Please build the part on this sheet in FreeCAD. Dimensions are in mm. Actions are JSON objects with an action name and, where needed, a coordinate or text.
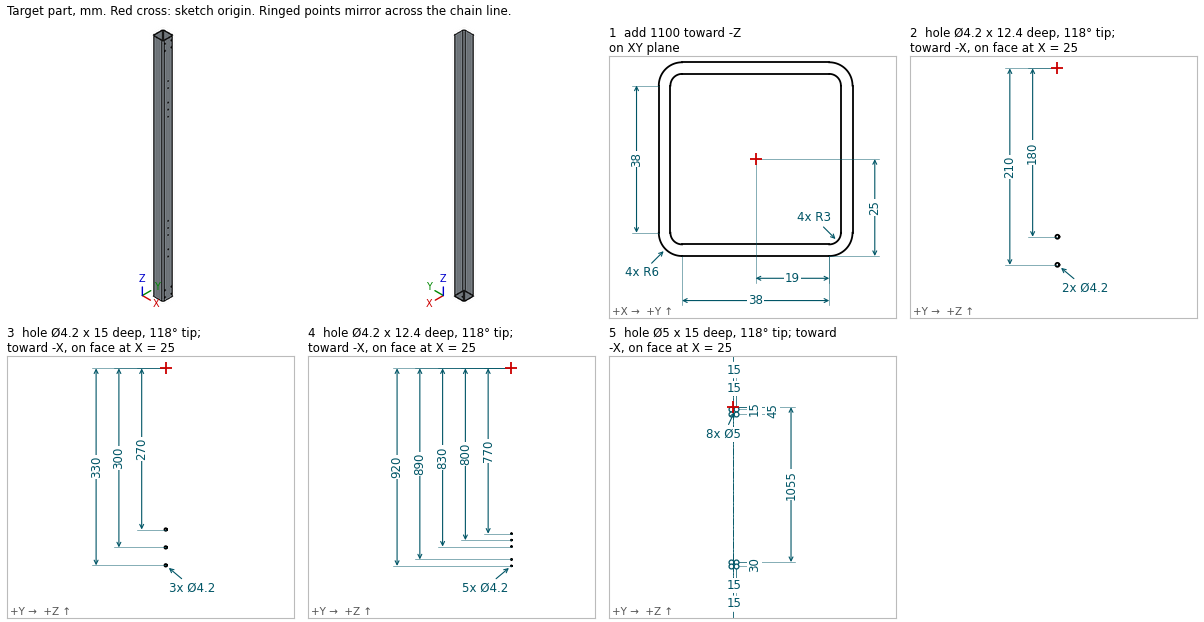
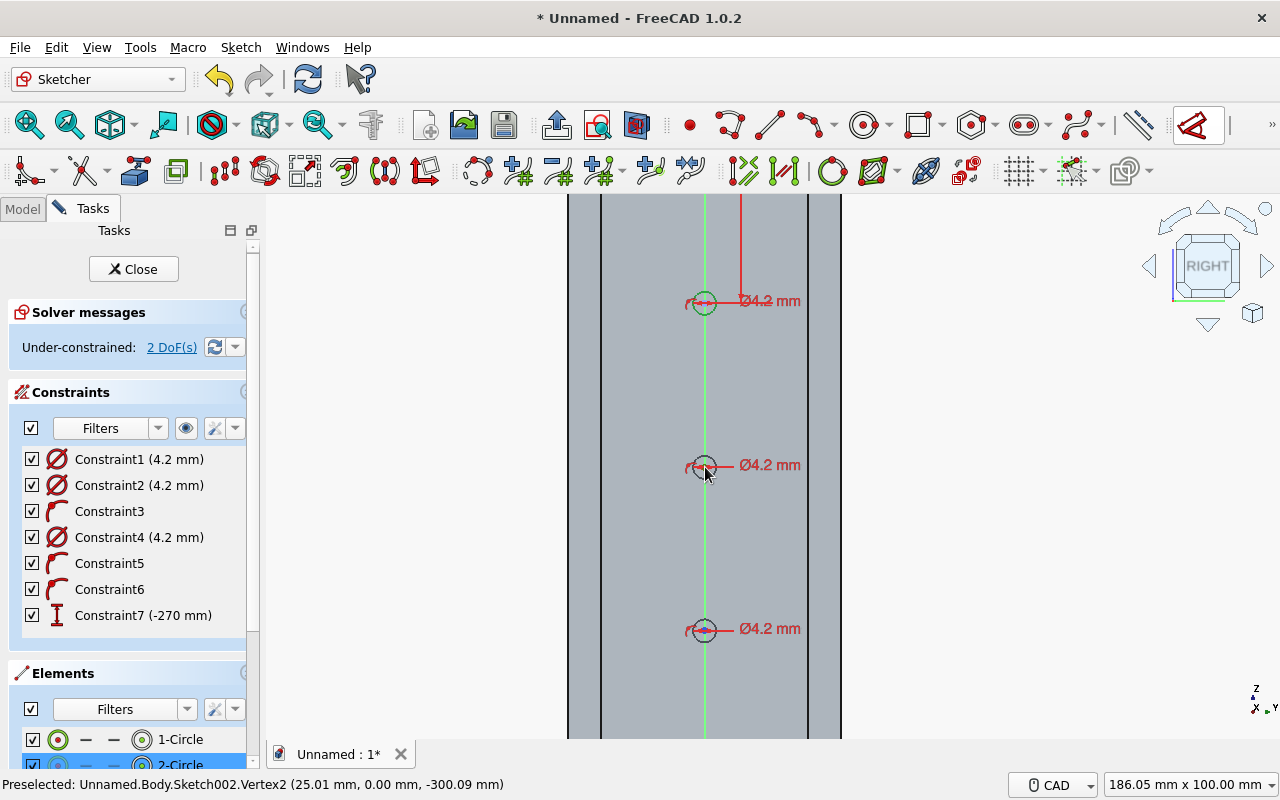
{"action": "key", "text": "i"}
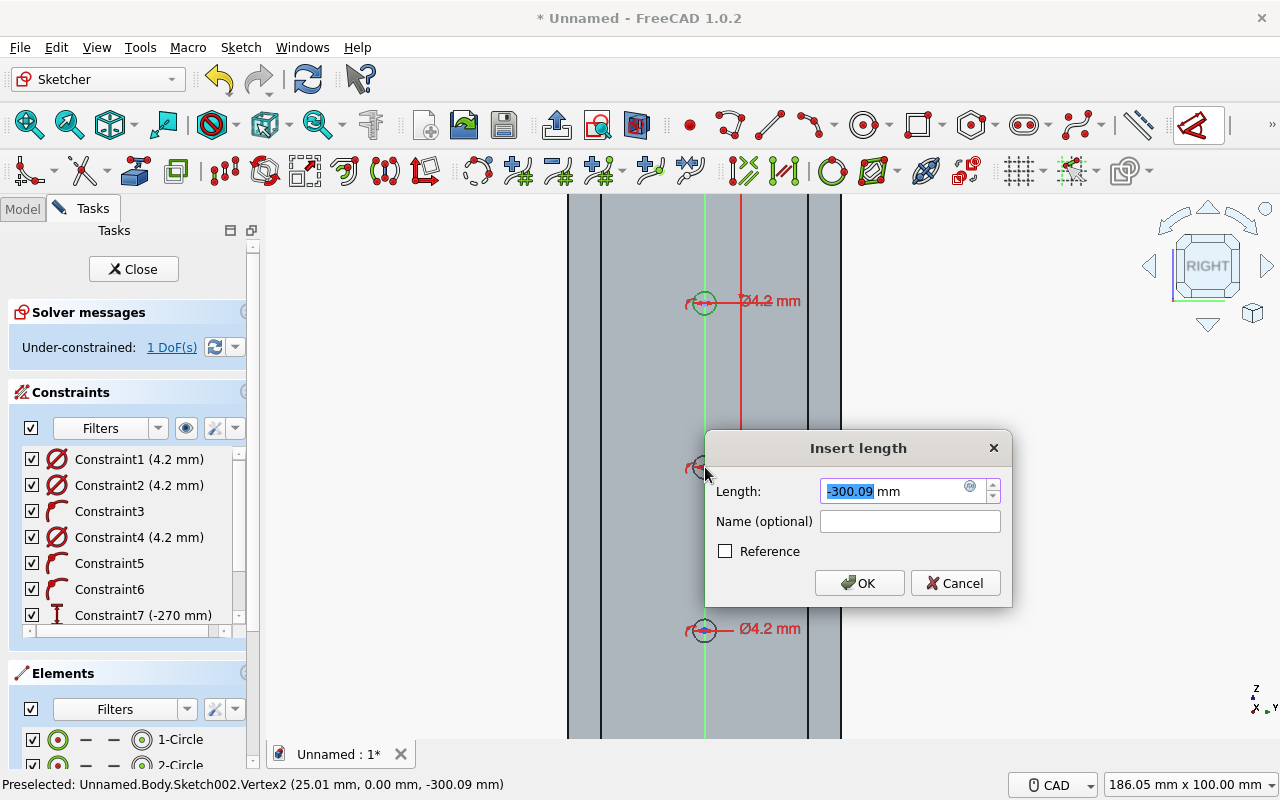
{"action": "type", "text": "-300"}
{"action": "key", "text": "Return"}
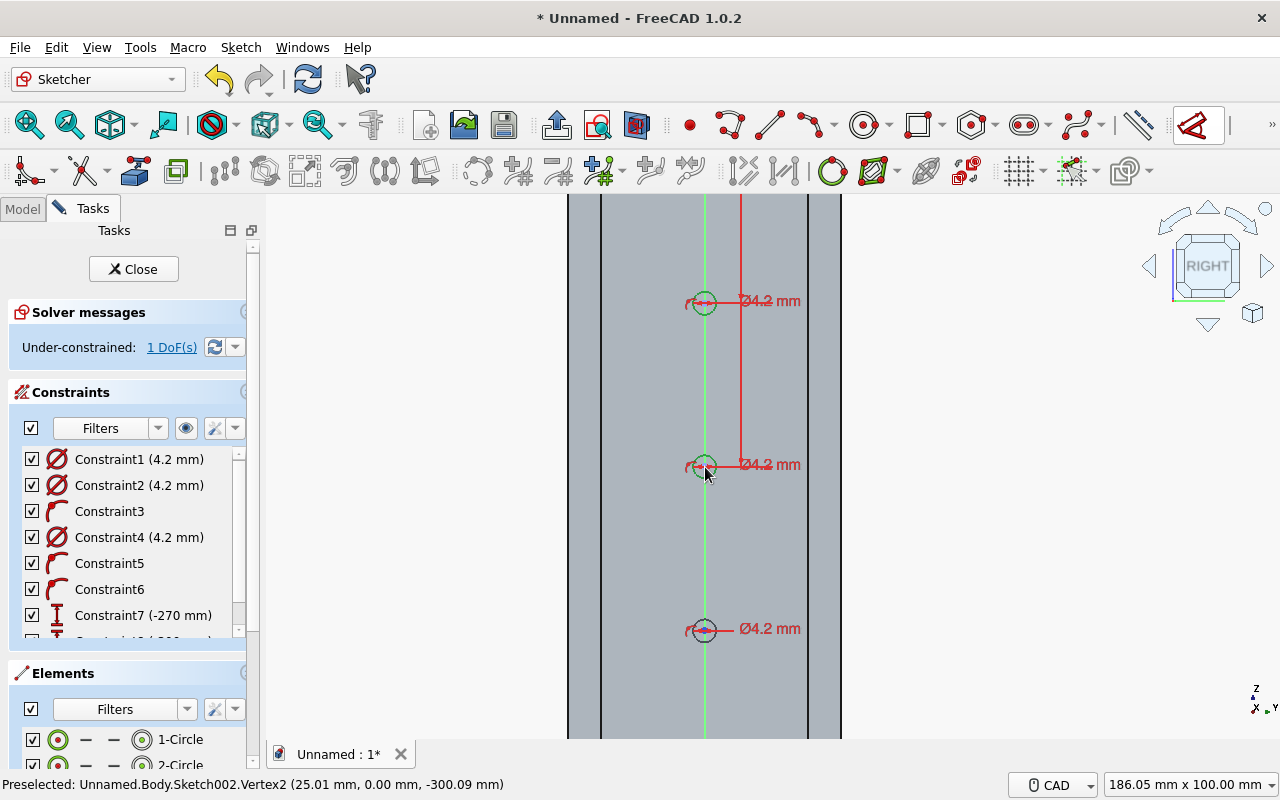
{"action": "left_click", "coordinate": [705, 631]}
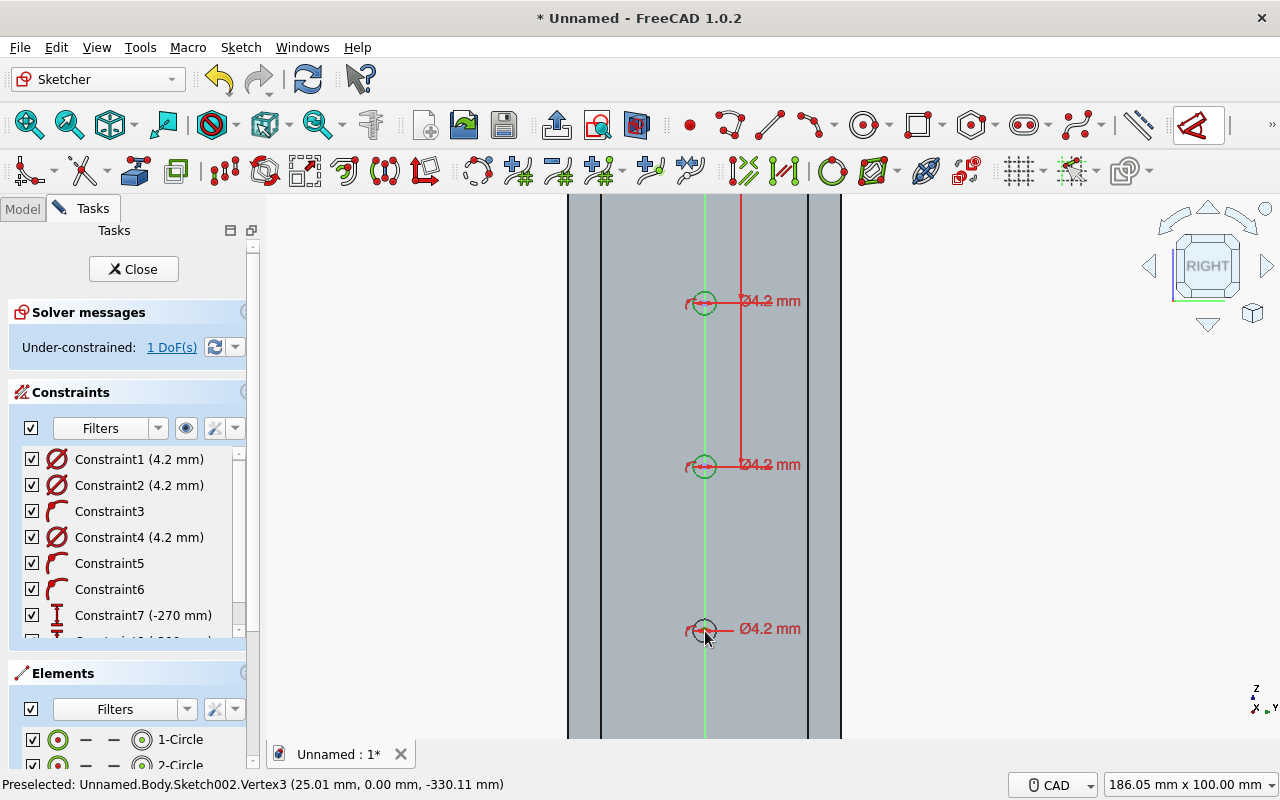
{"action": "left_click", "coordinate": [1218, 126]}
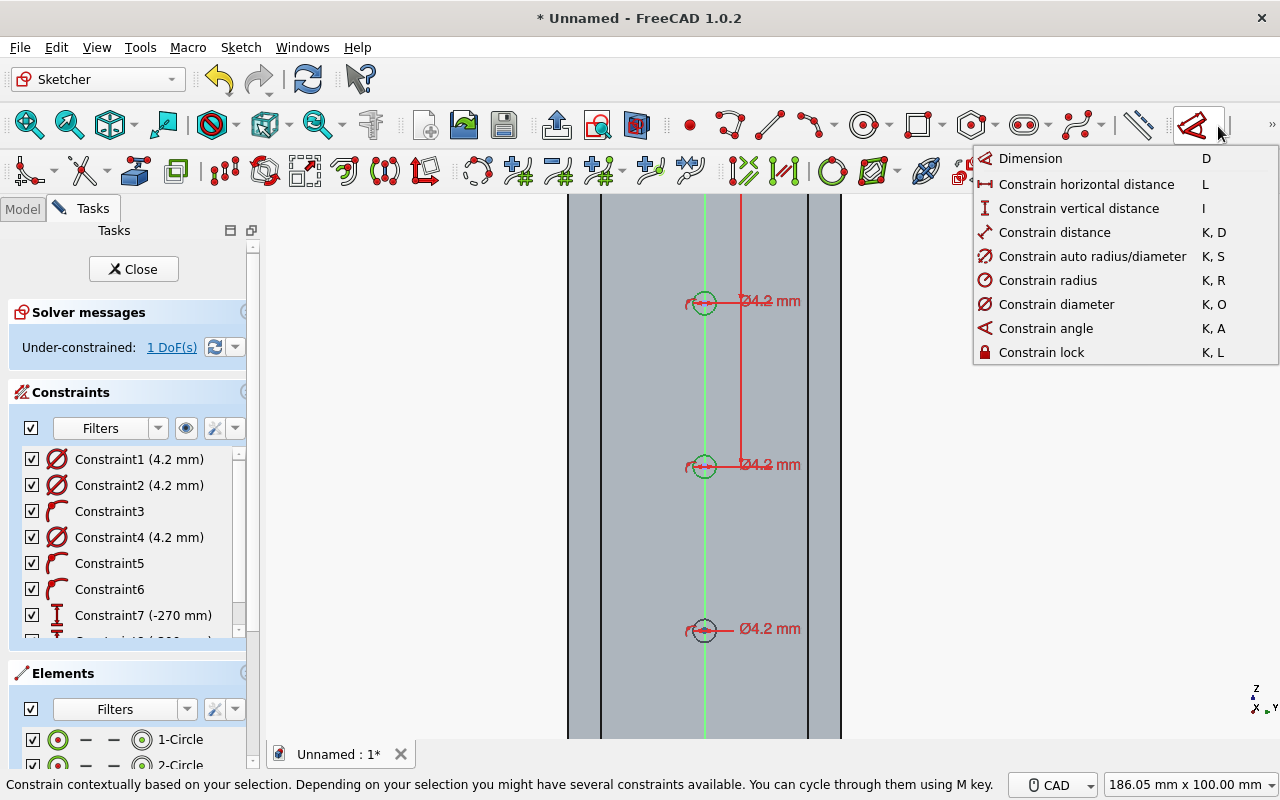
{"action": "left_click", "coordinate": [1126, 208]}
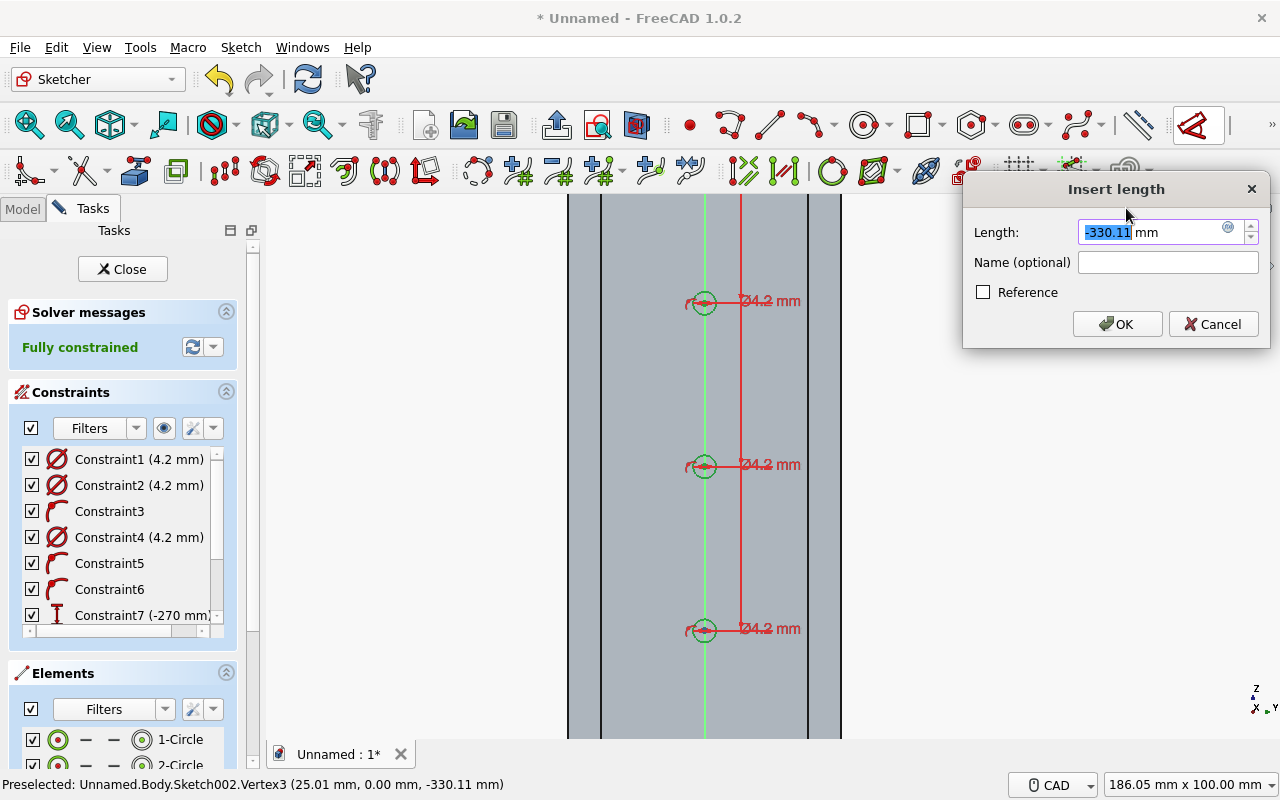
{"action": "type", "text": "-330"}
{"action": "key", "text": "Return"}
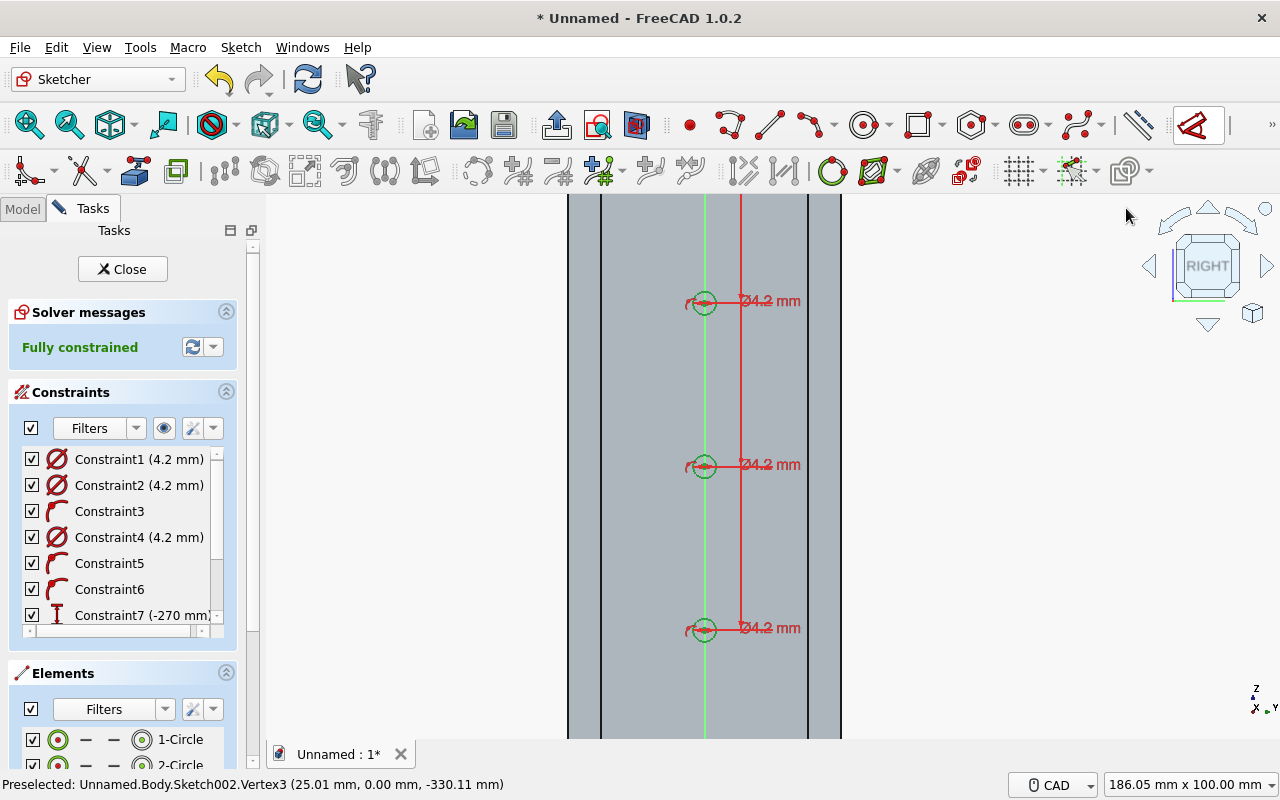
{"action": "left_click", "coordinate": [123, 269]}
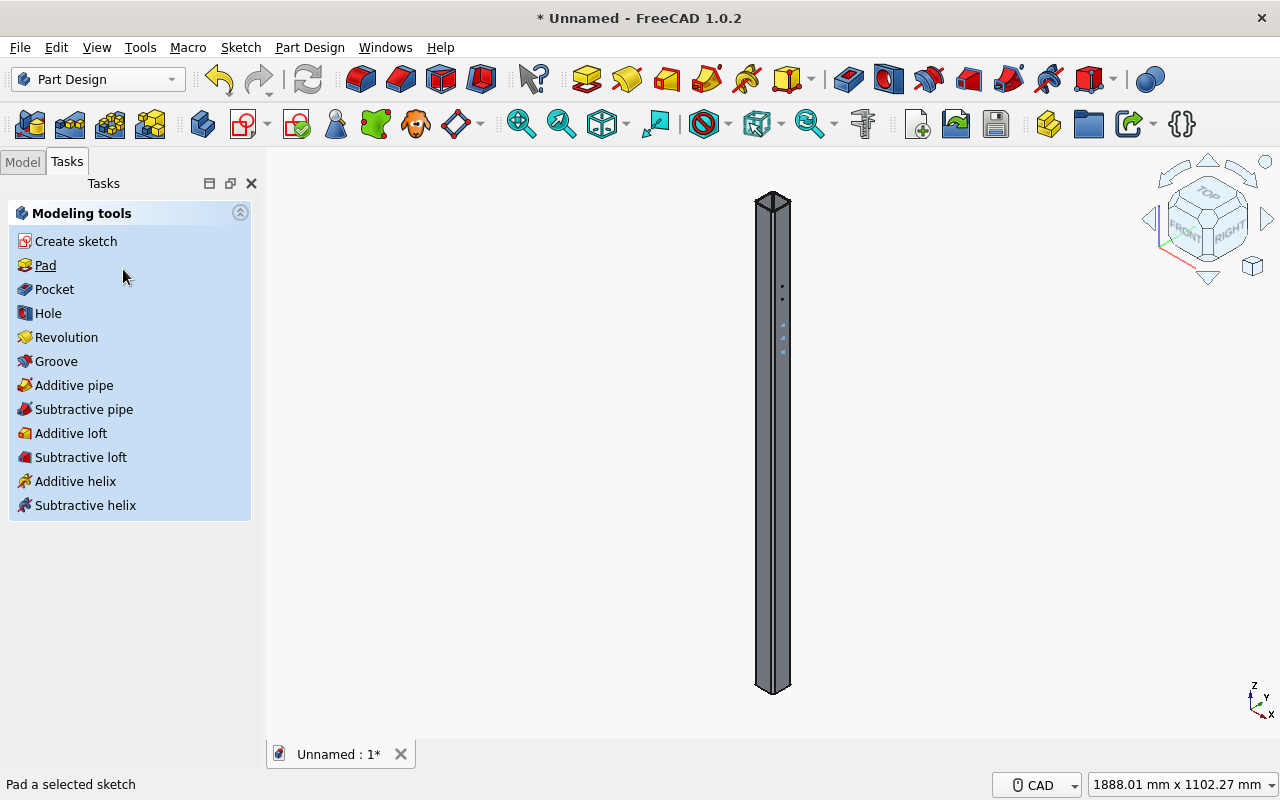
{"action": "left_click", "coordinate": [890, 80]}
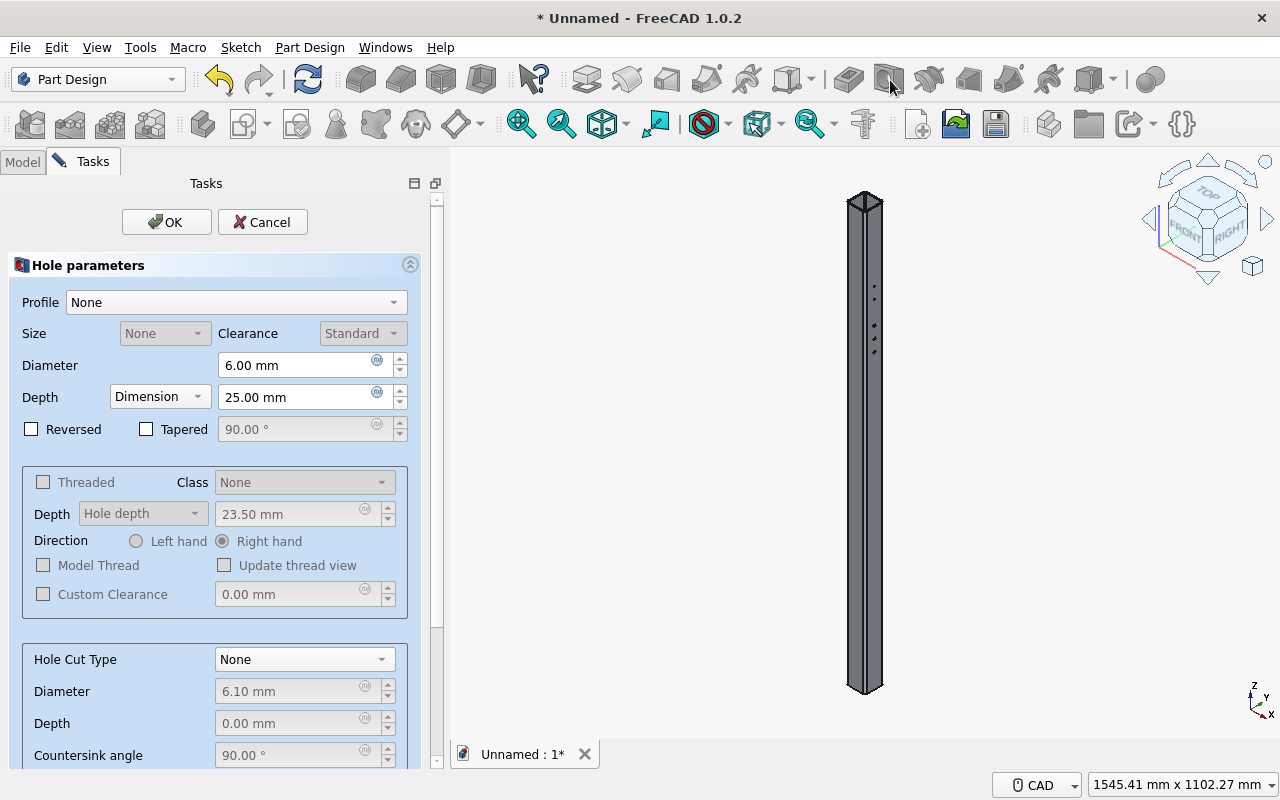
{"action": "triple_click", "coordinate": [305, 365]}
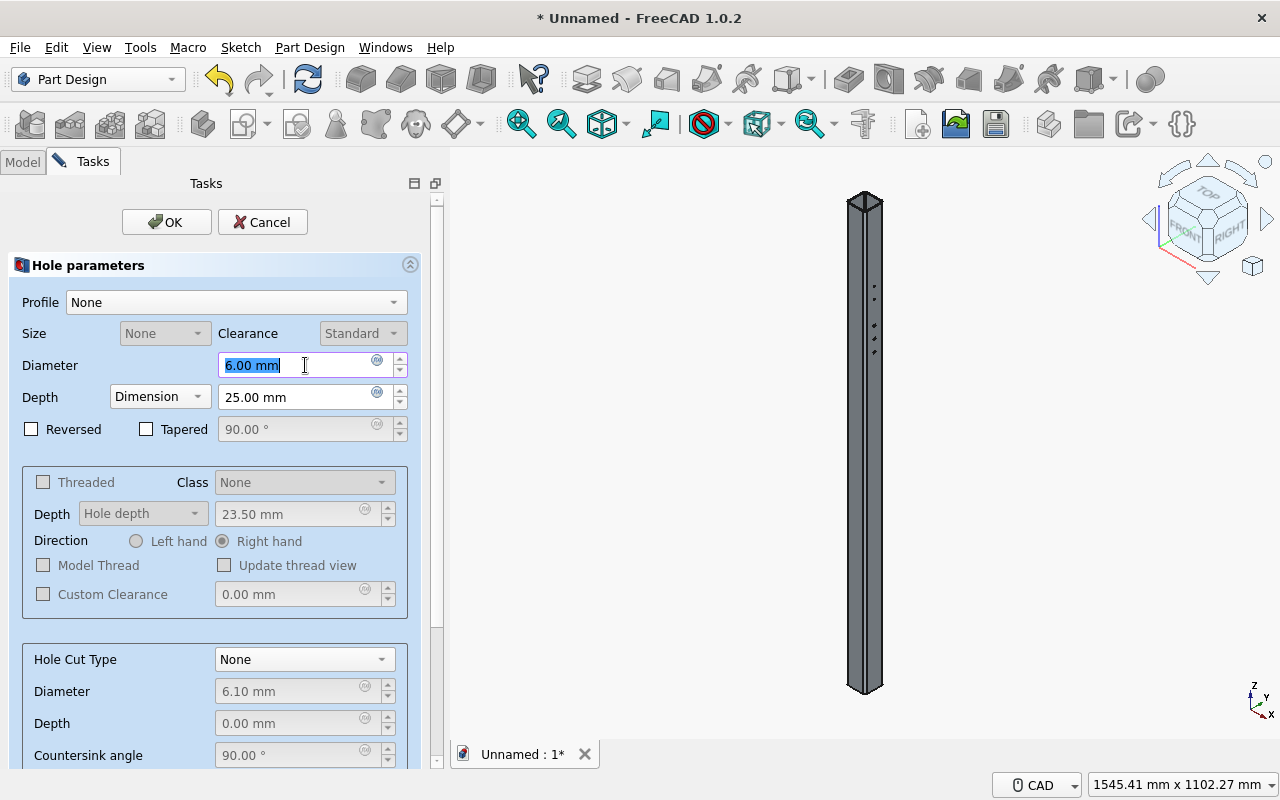
{"action": "type", "text": "4.2"}
{"action": "key", "text": "Tab"}